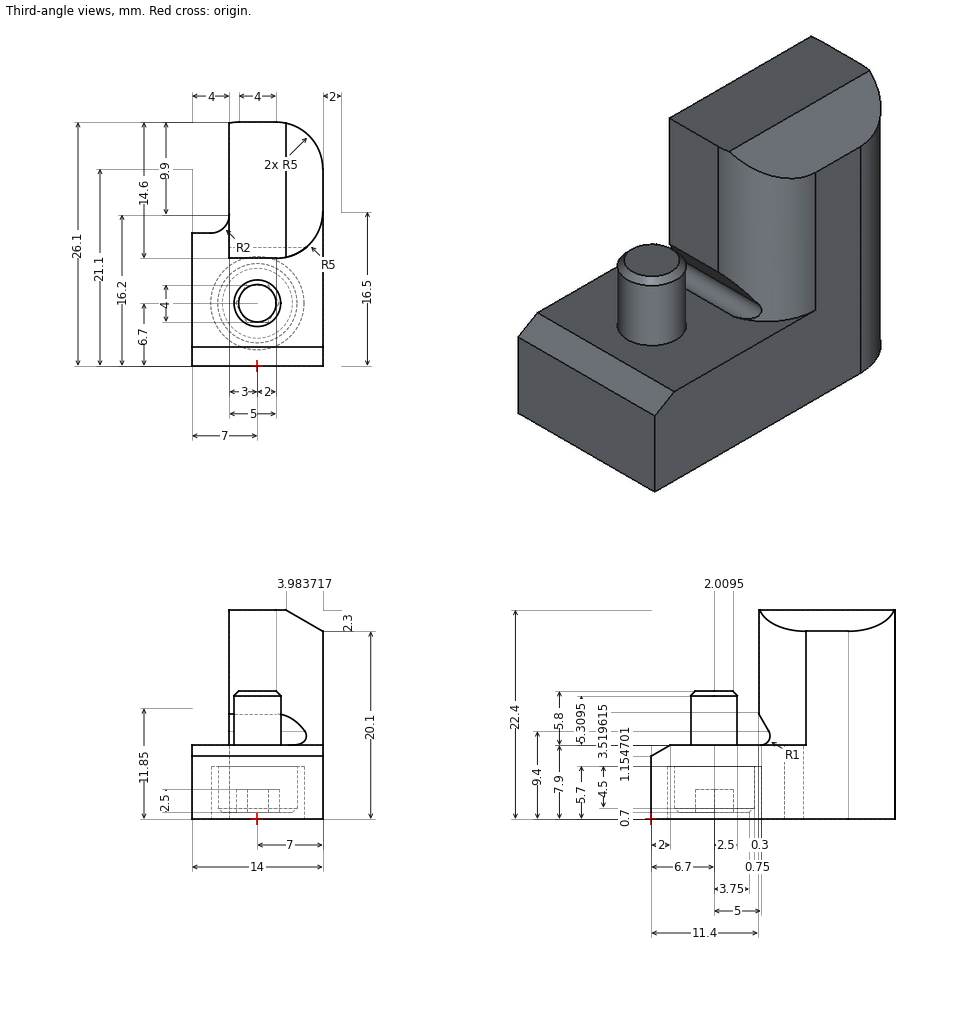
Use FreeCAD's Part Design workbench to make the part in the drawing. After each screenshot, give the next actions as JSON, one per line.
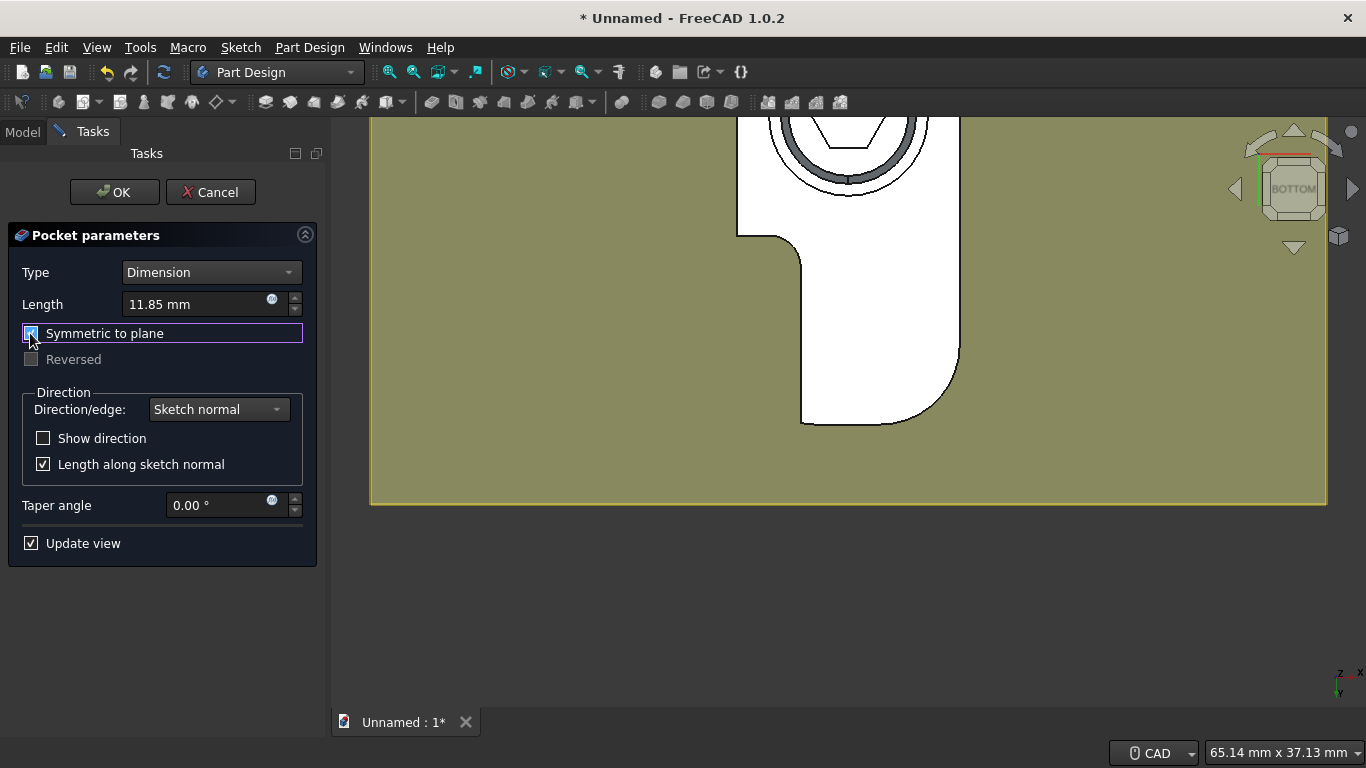
{"action": "left_click", "coordinate": [115, 192]}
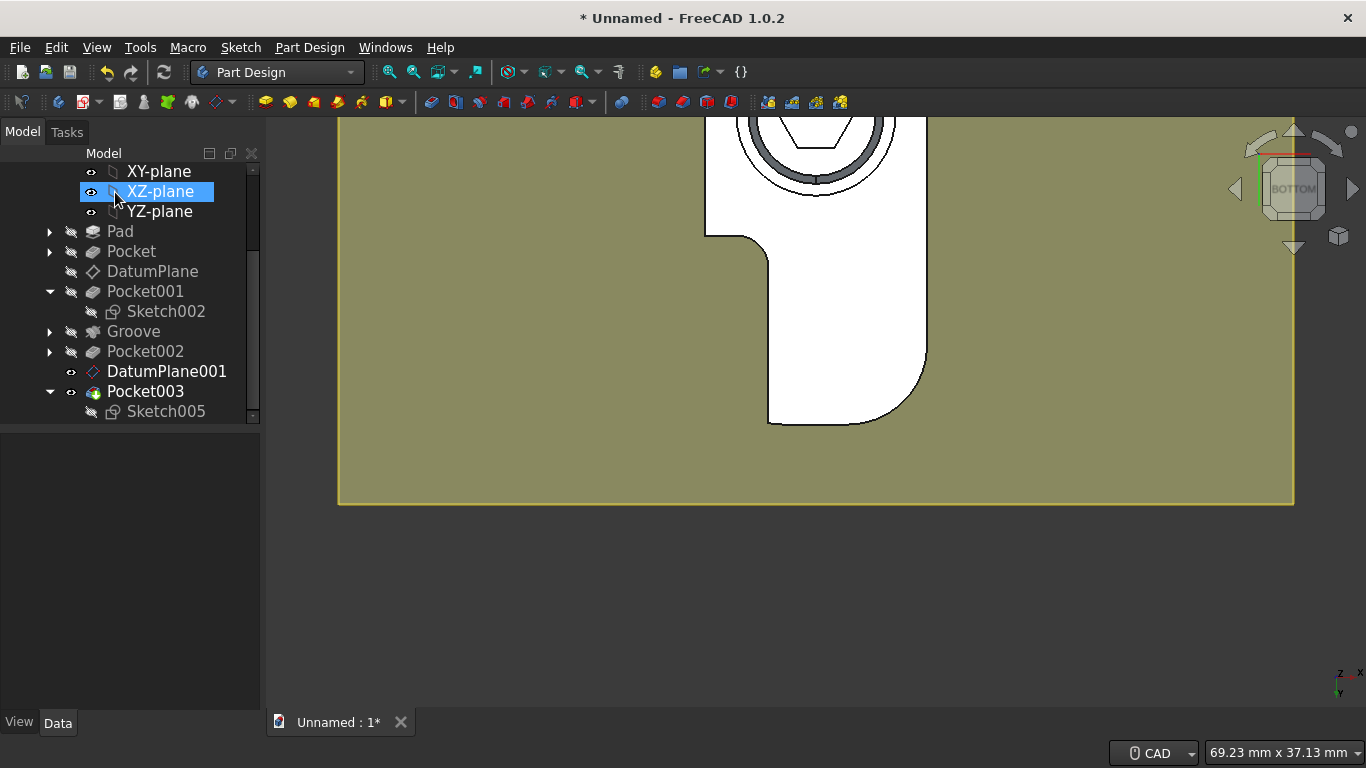
{"action": "left_click", "coordinate": [116, 372]}
{"action": "key", "text": "space"}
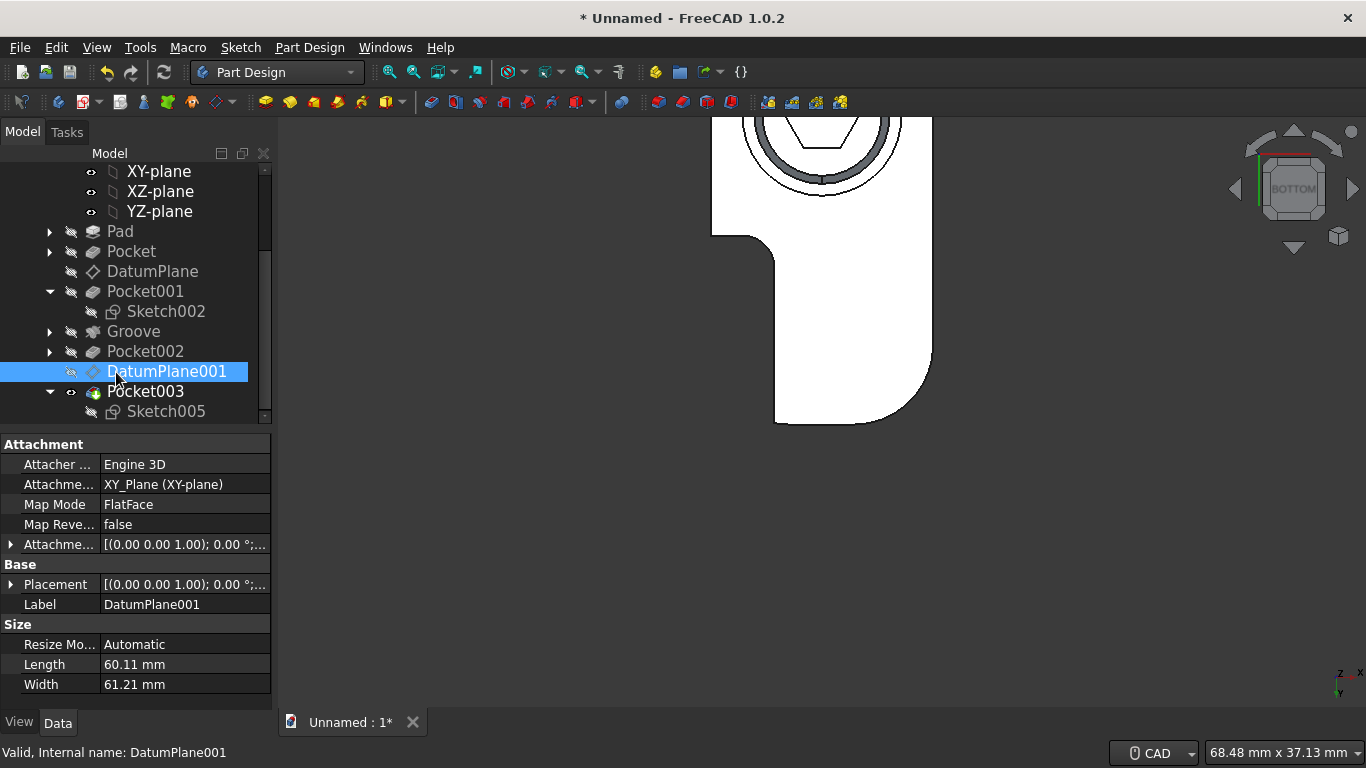
{"action": "left_click", "coordinate": [390, 72]}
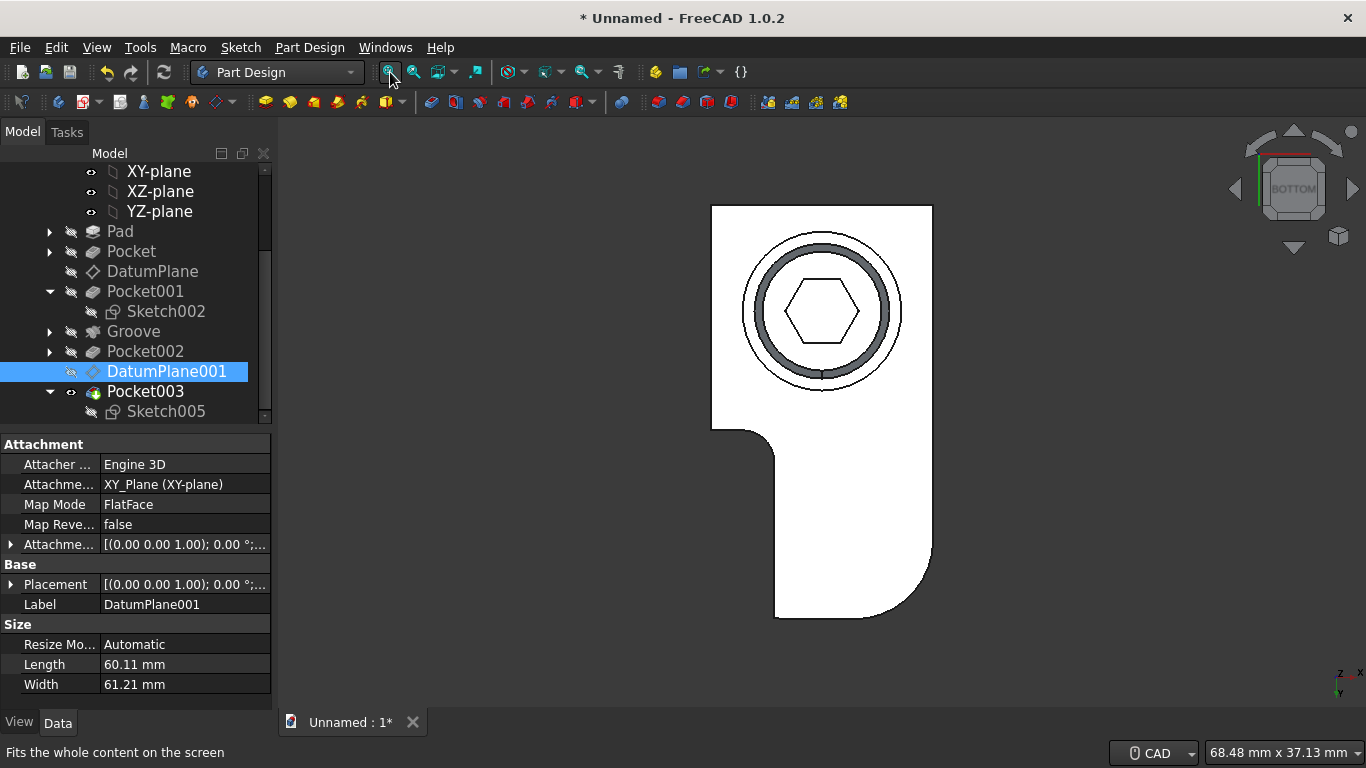
{"action": "left_click", "coordinate": [318, 667]}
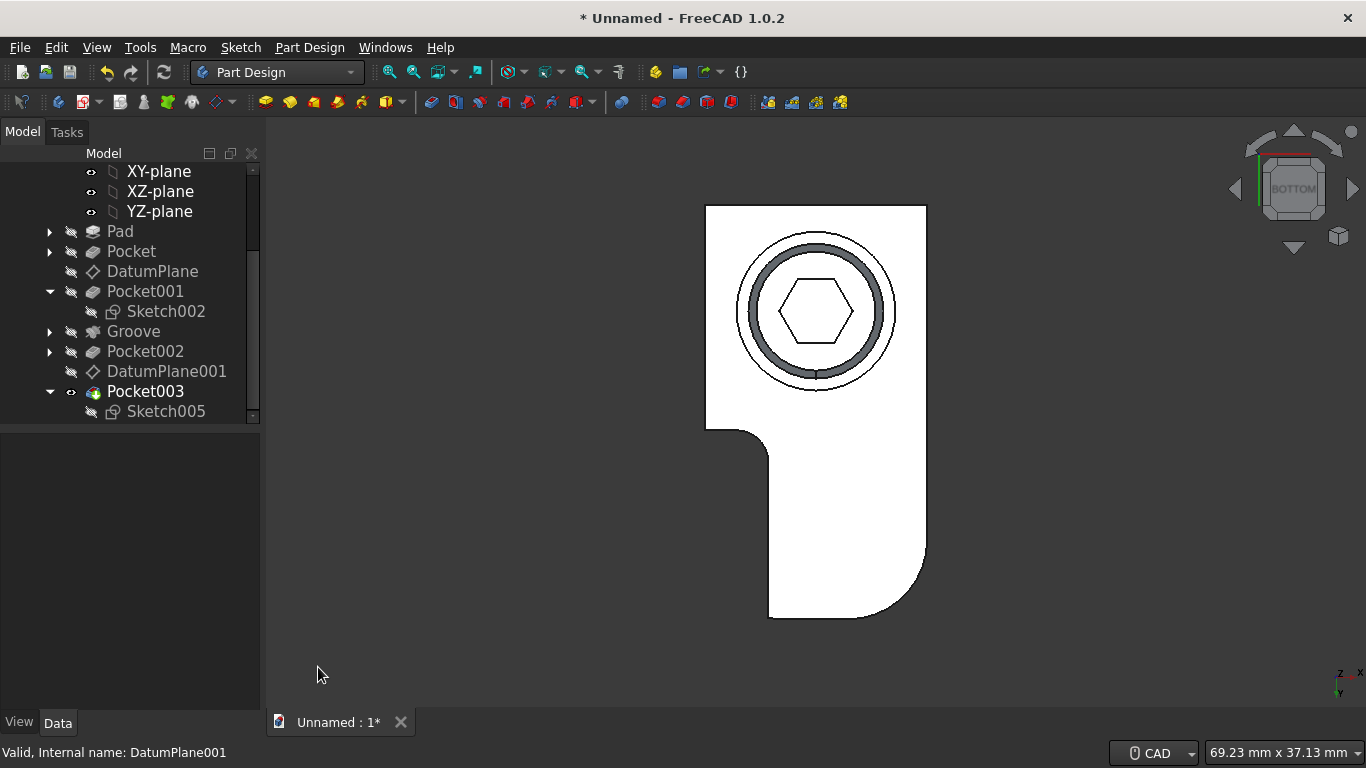
{"action": "left_click", "coordinate": [84, 102]}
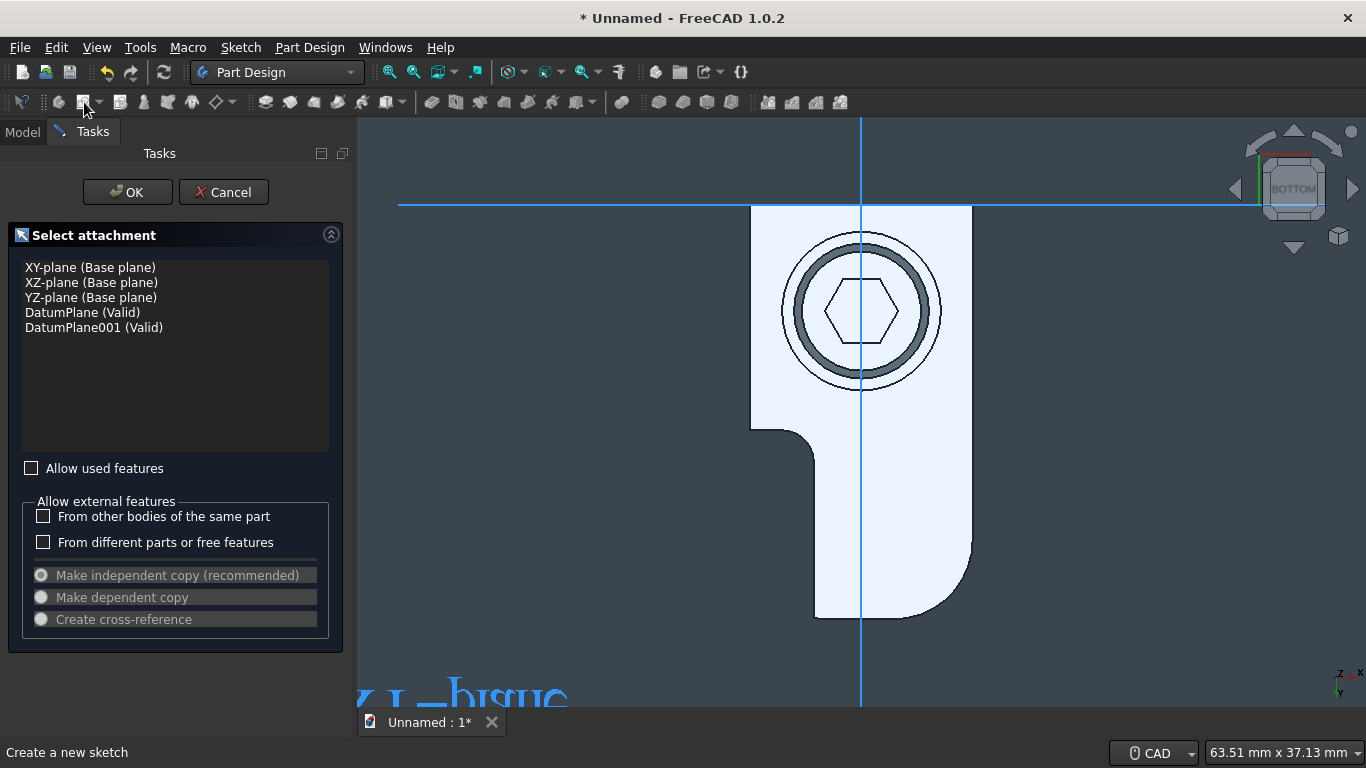
{"action": "left_click", "coordinate": [82, 298]}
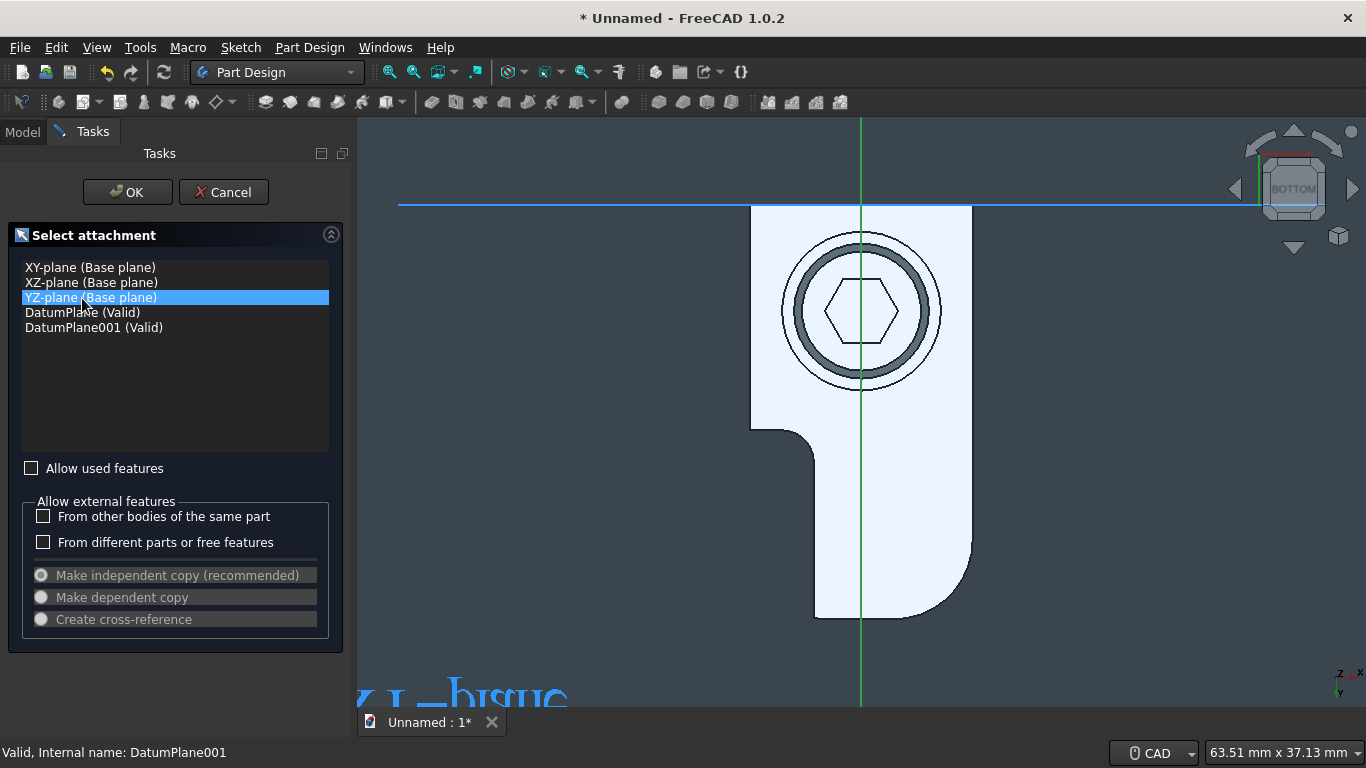
{"action": "left_click", "coordinate": [128, 192]}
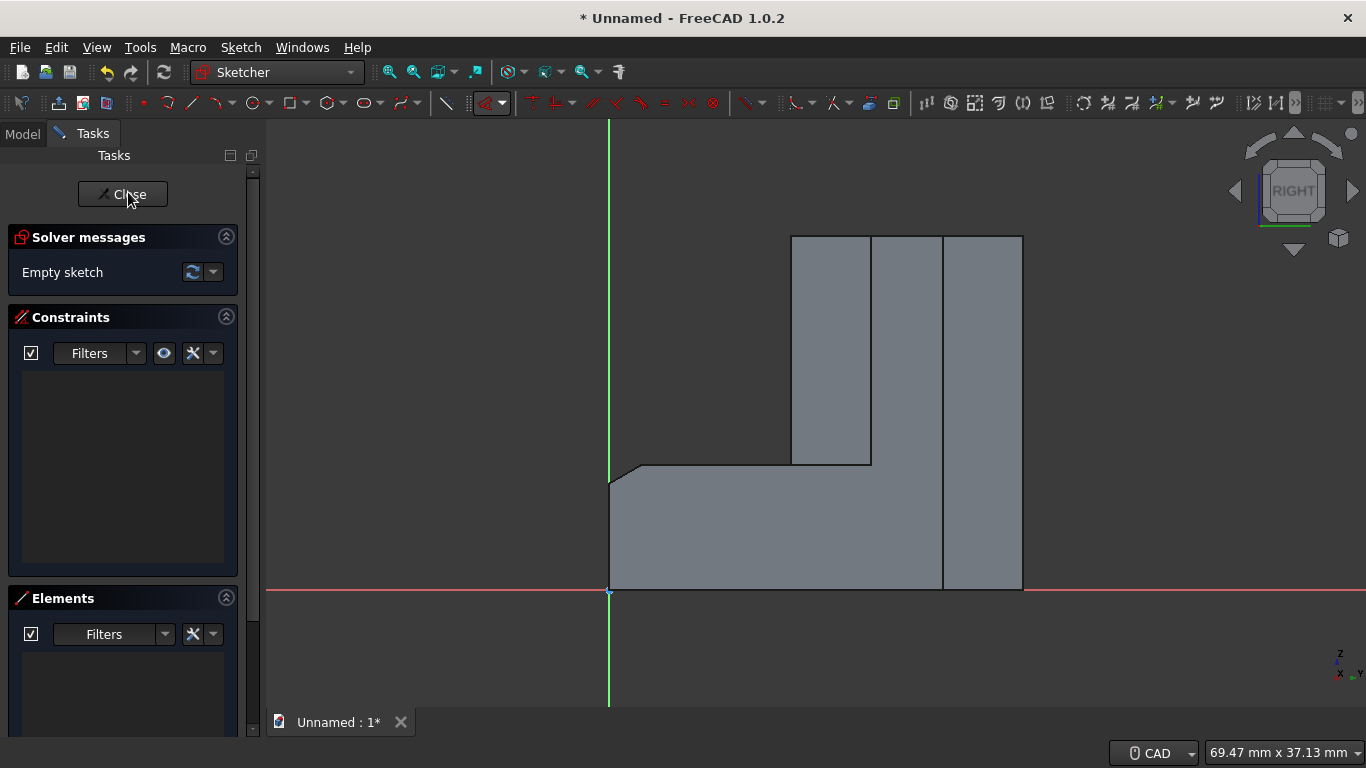
{"action": "left_click", "coordinate": [108, 104]}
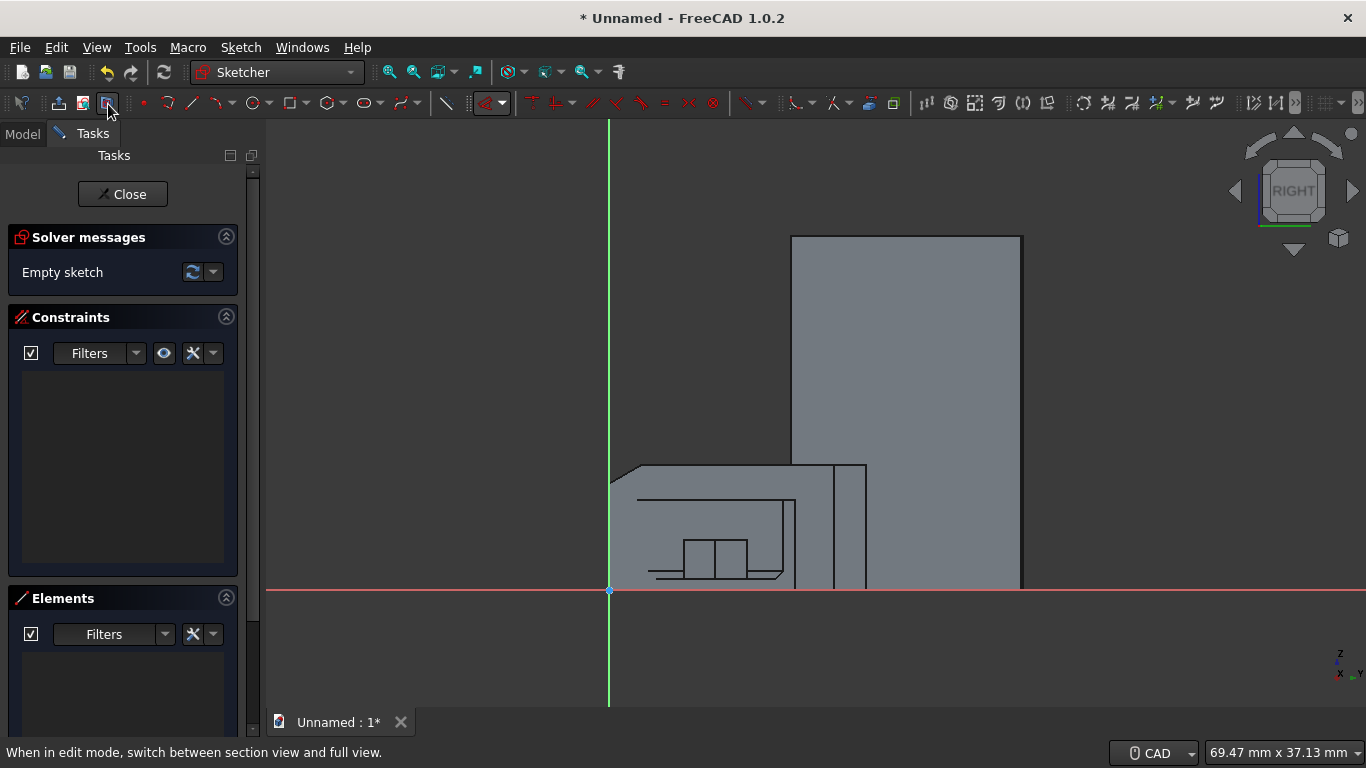
{"action": "scroll", "coordinate": [807, 441], "scroll_direction": "up", "scroll_amount": 10}